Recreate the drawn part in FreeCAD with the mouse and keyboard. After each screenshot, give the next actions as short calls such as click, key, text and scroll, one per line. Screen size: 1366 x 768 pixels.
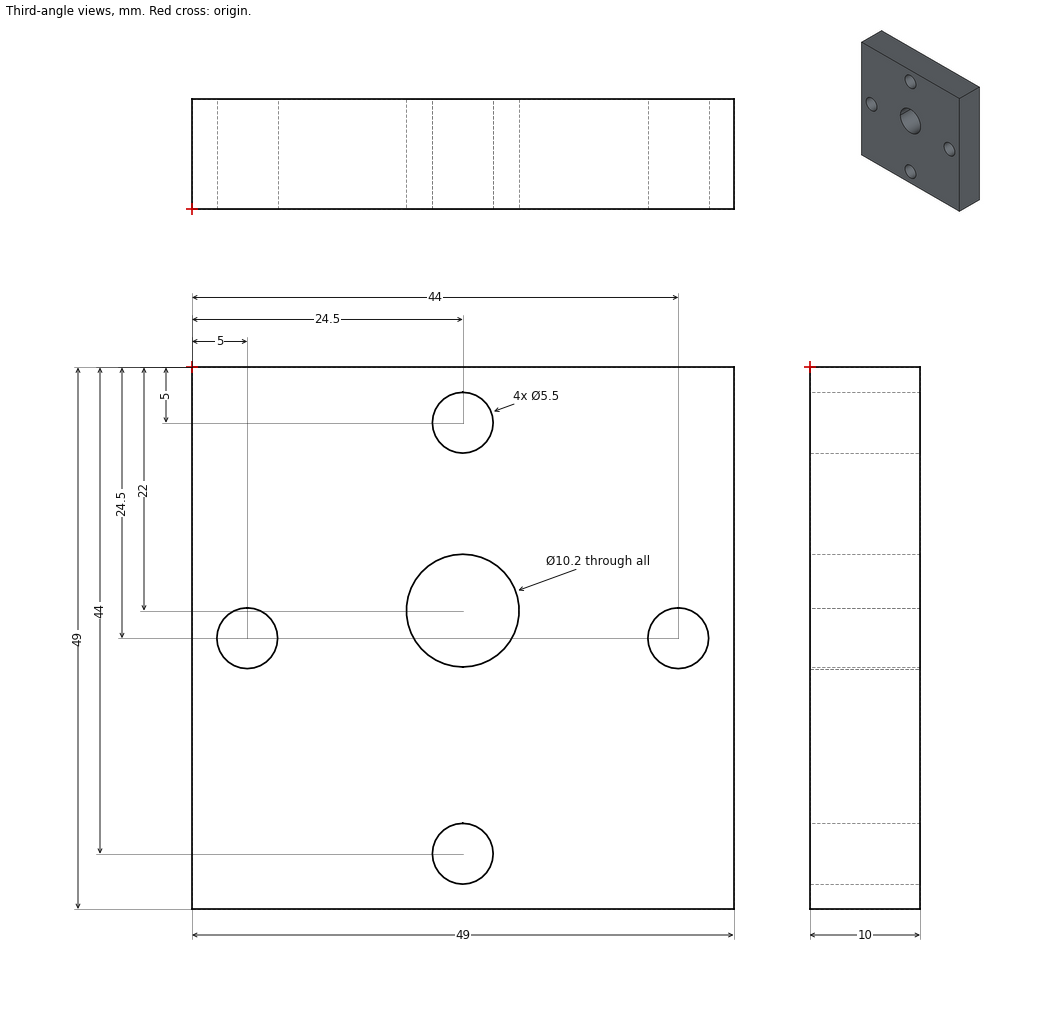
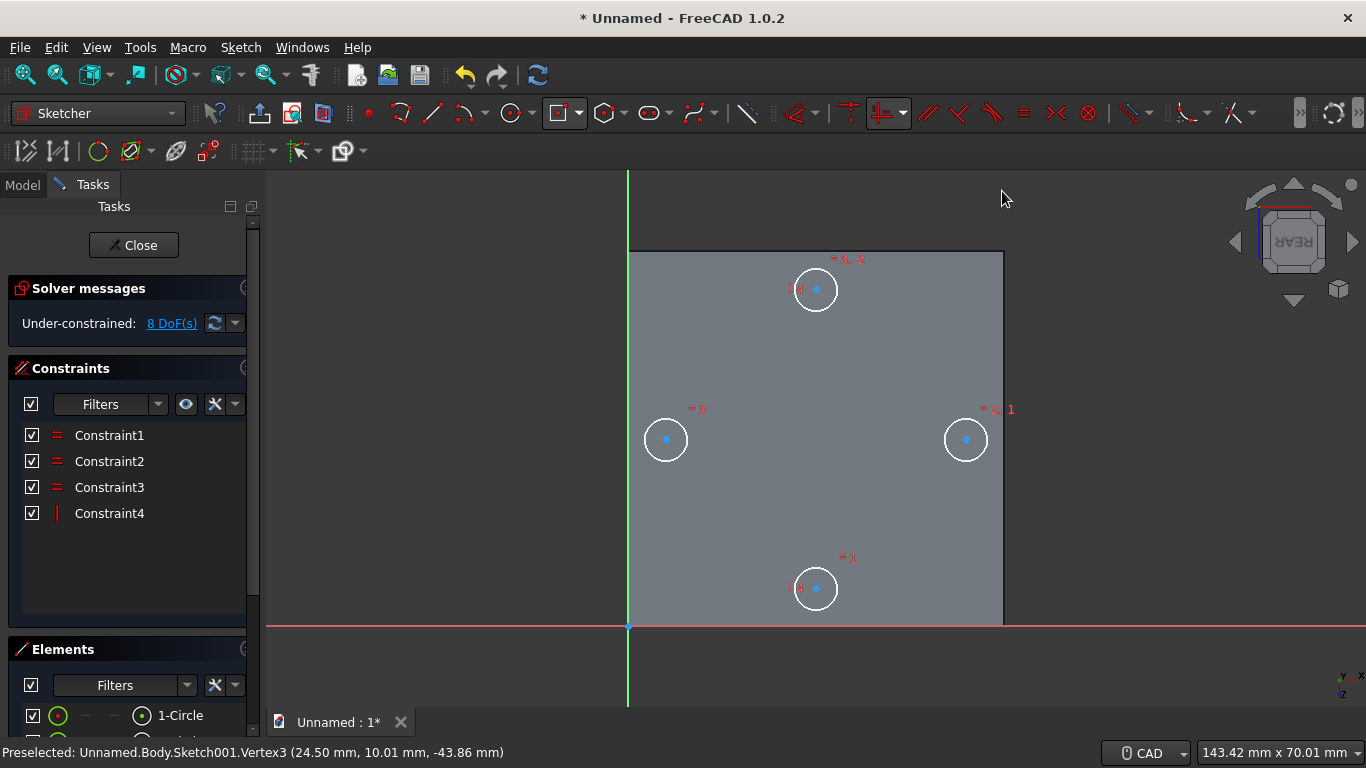
click(966, 440)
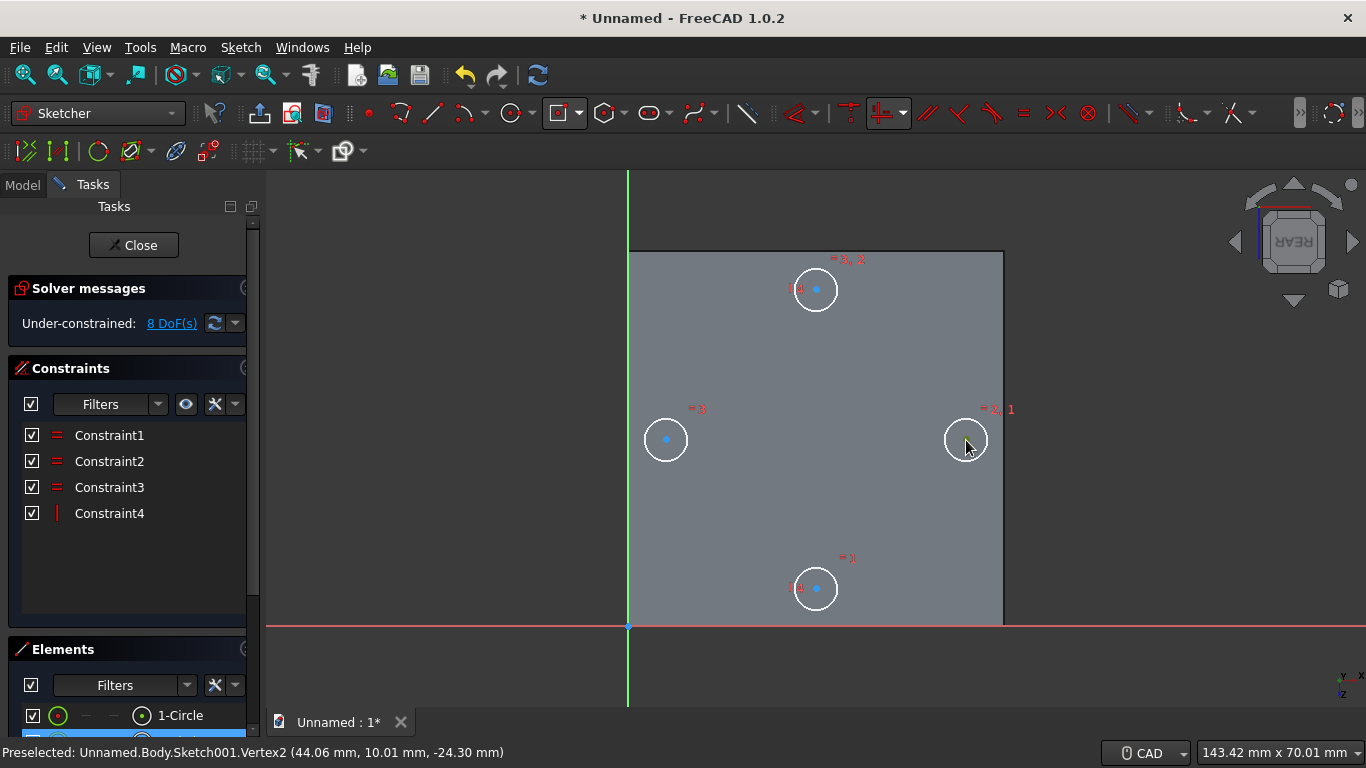
click(666, 440)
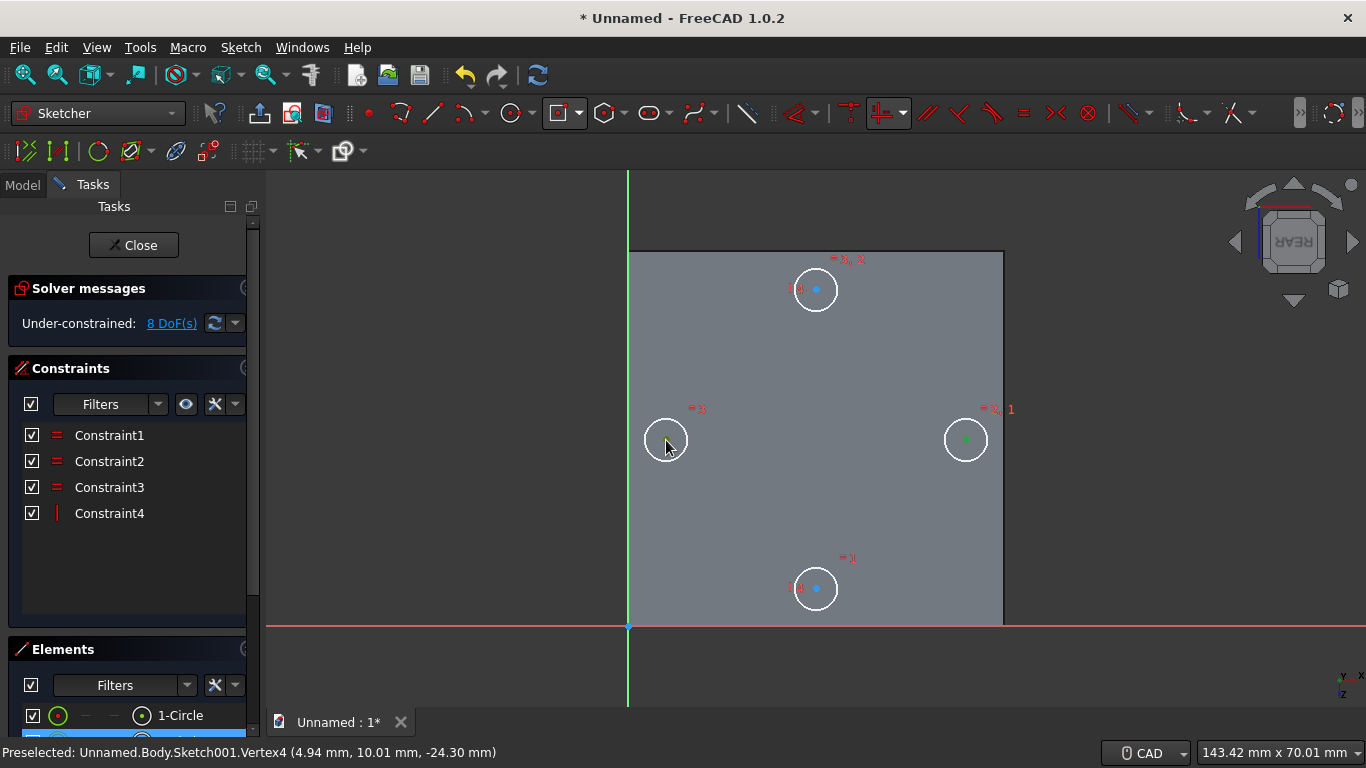
click(906, 114)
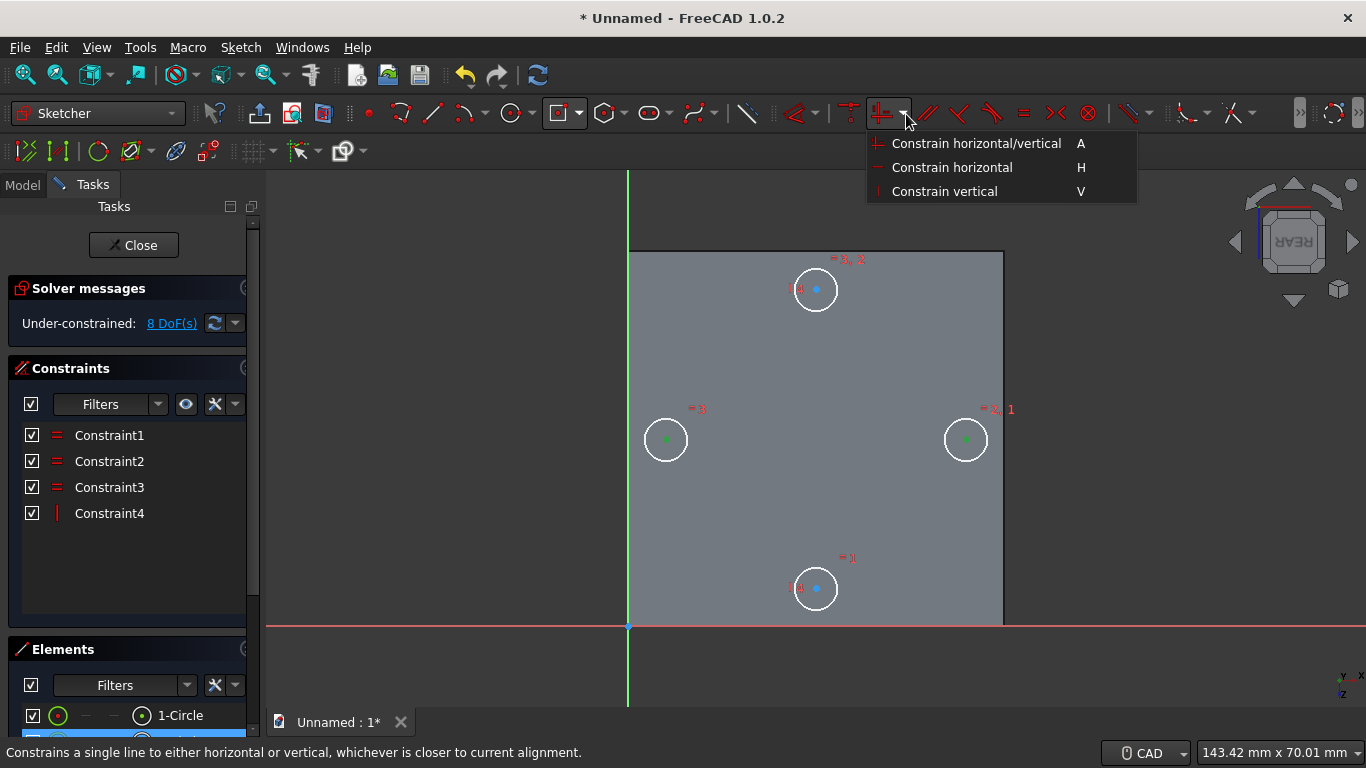
click(1002, 167)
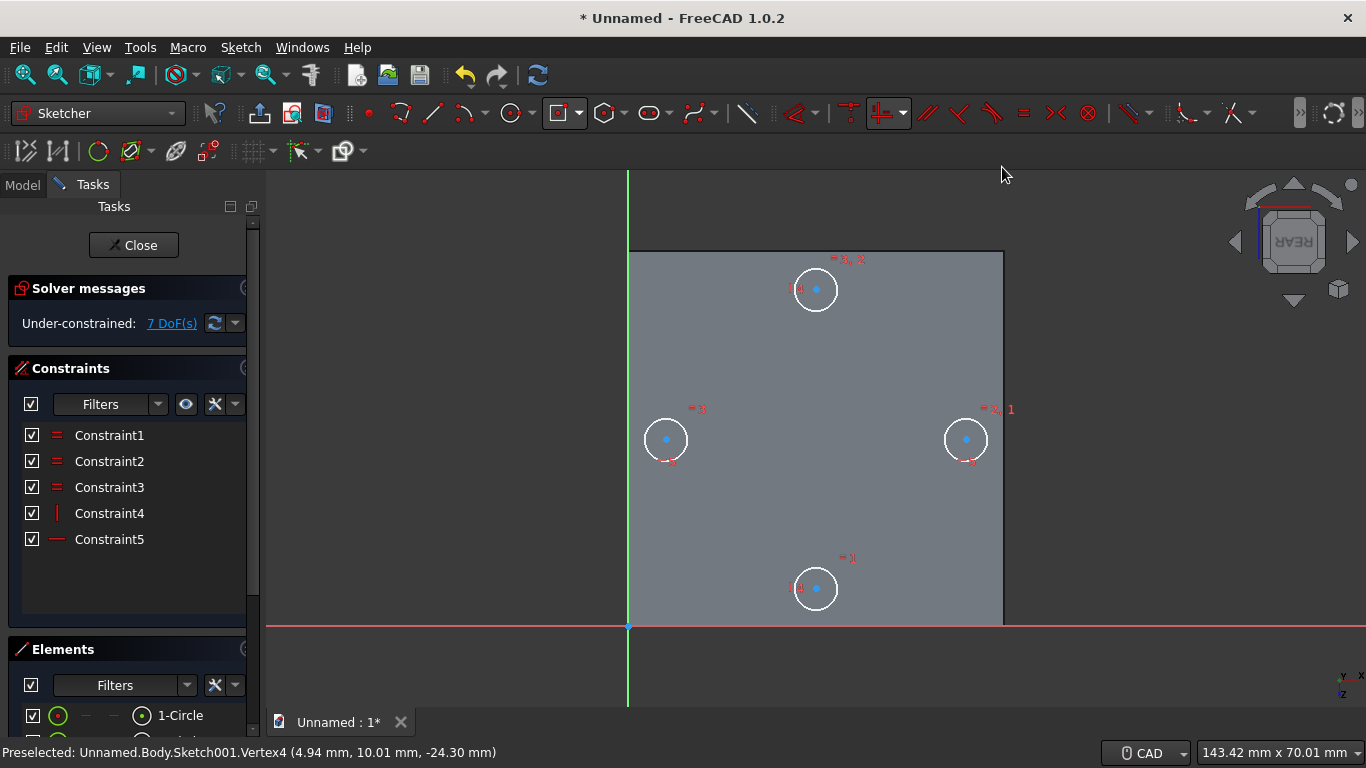
key(d)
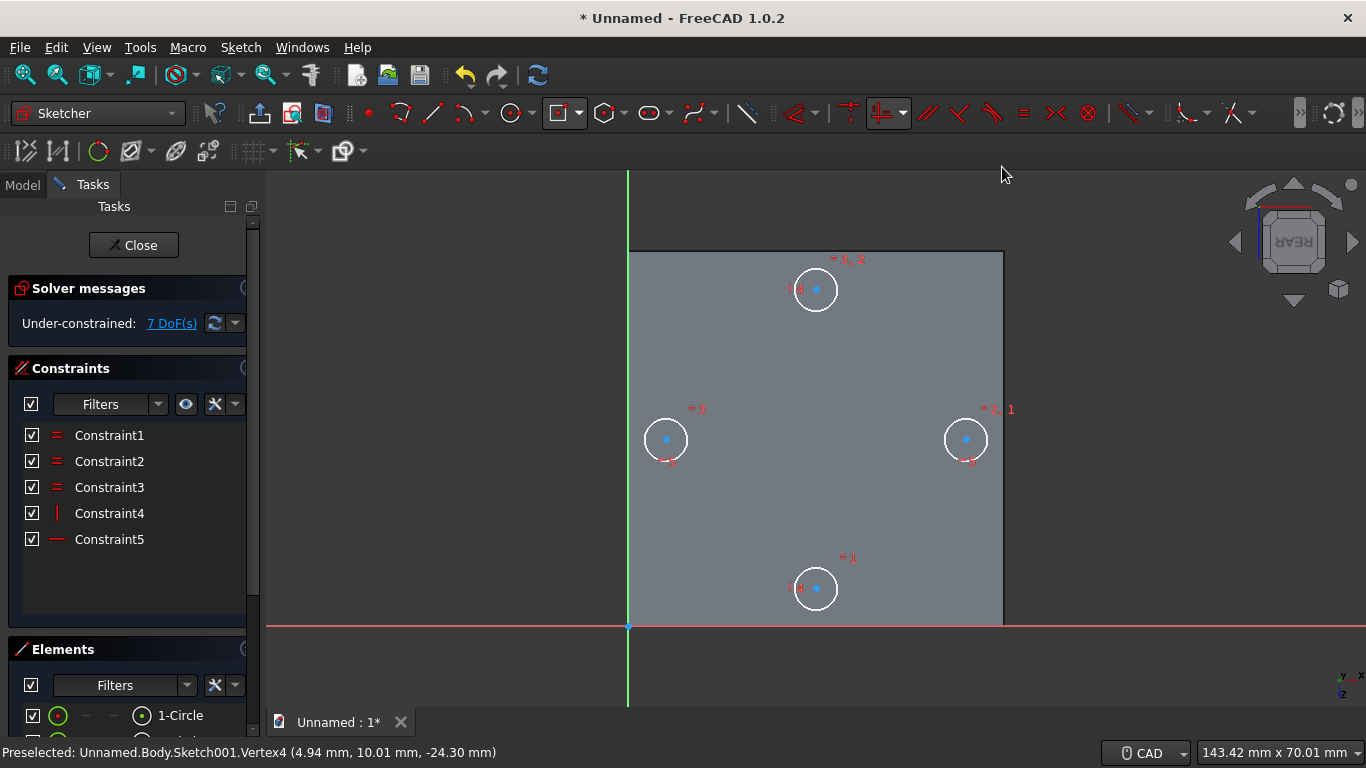
click(831, 574)
click(854, 551)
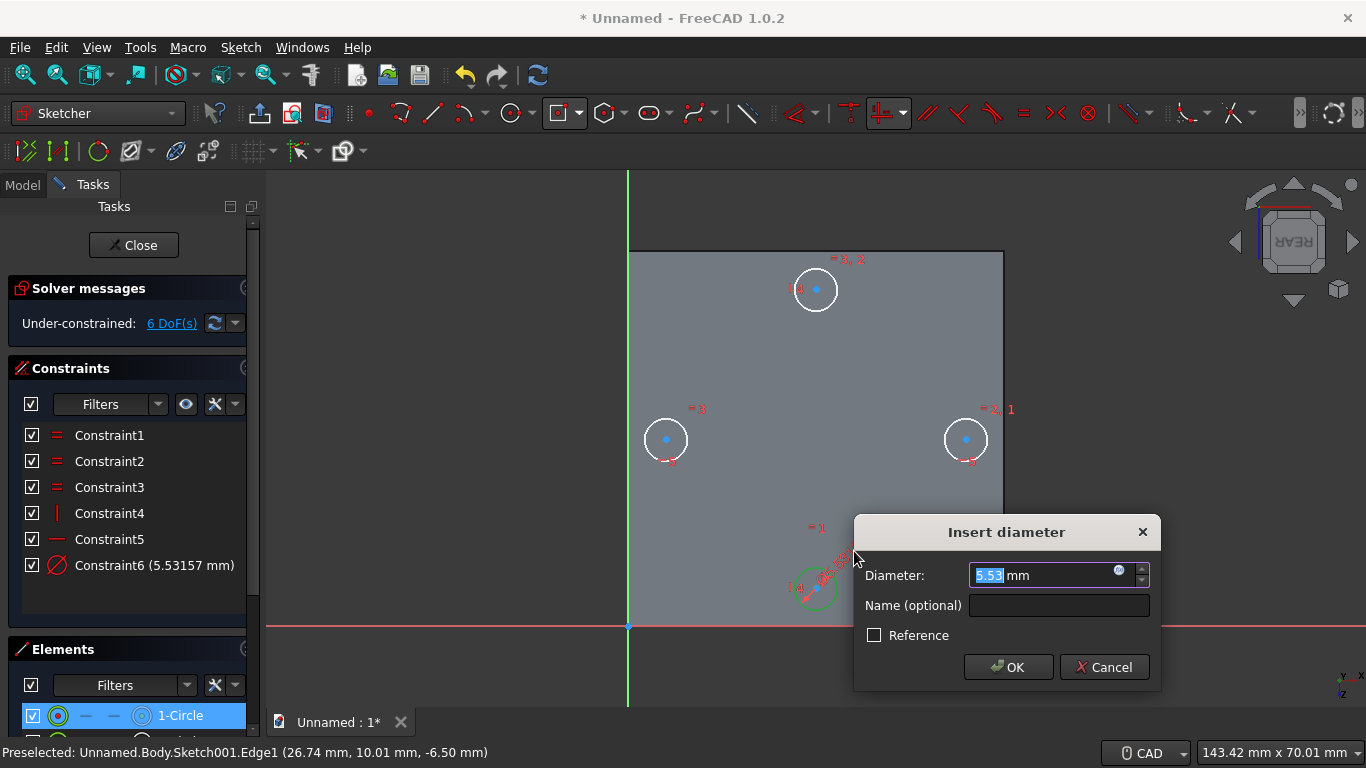
text(5.5)
key(Return)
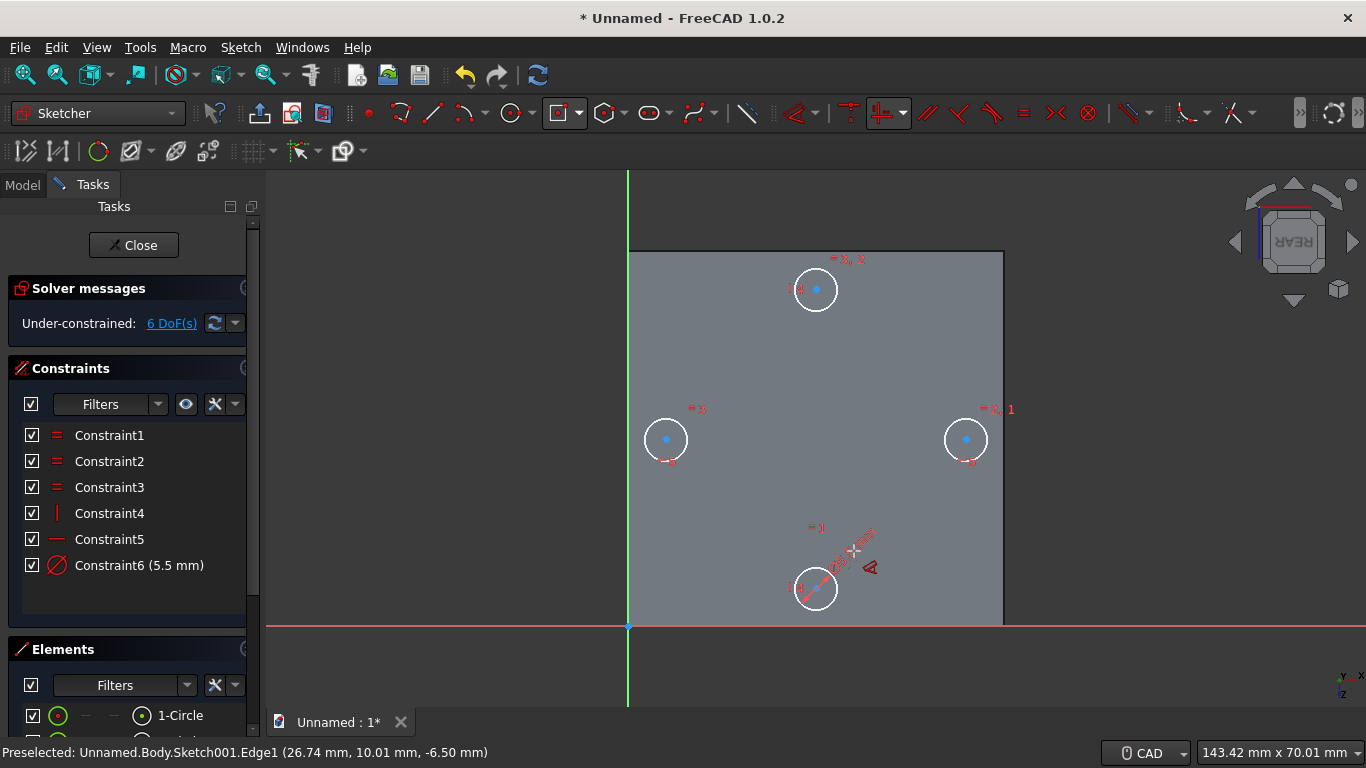
click(816, 589)
click(594, 608)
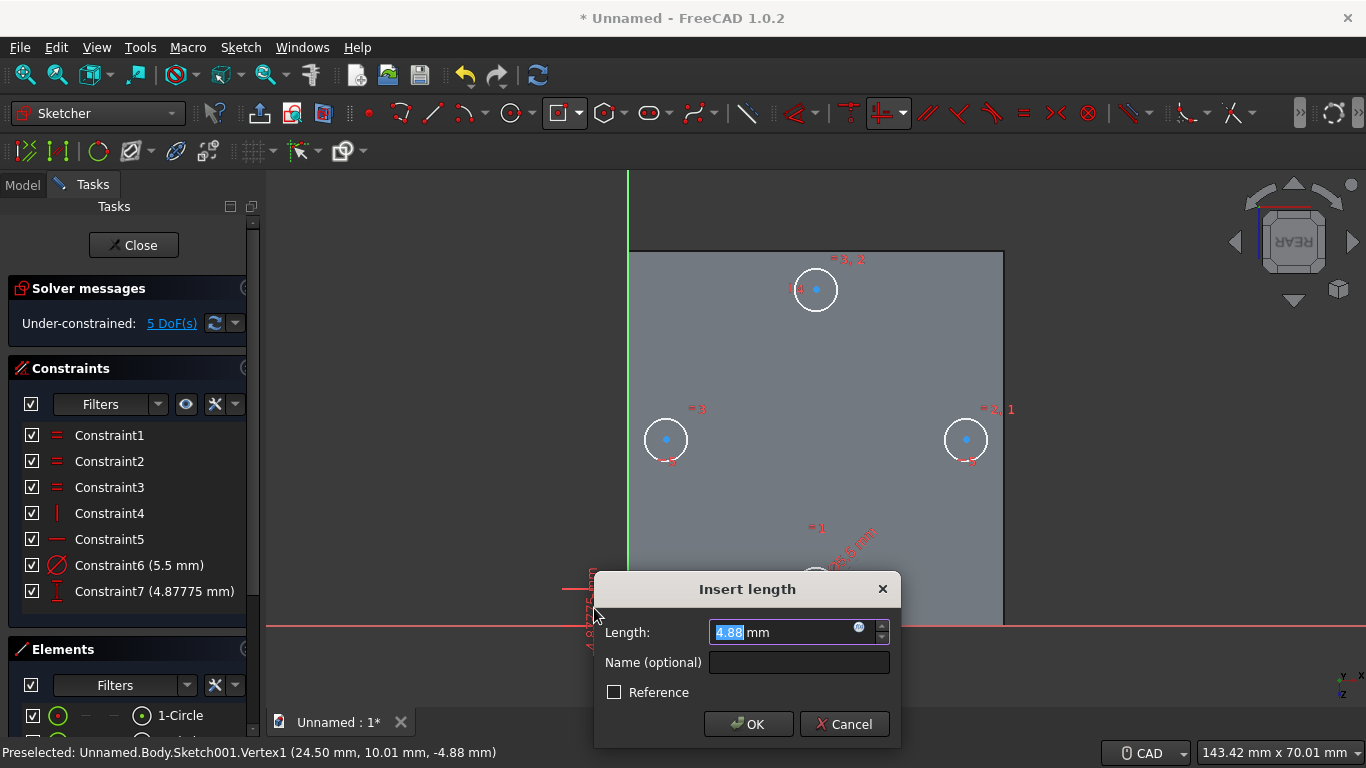
text(5)
key(Return)